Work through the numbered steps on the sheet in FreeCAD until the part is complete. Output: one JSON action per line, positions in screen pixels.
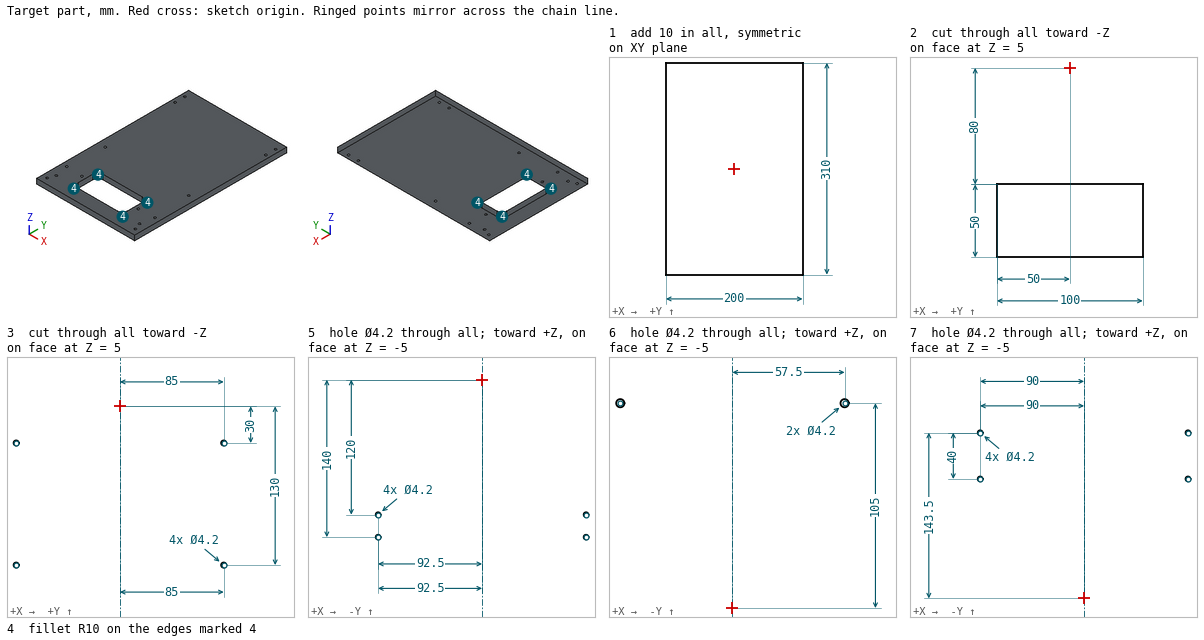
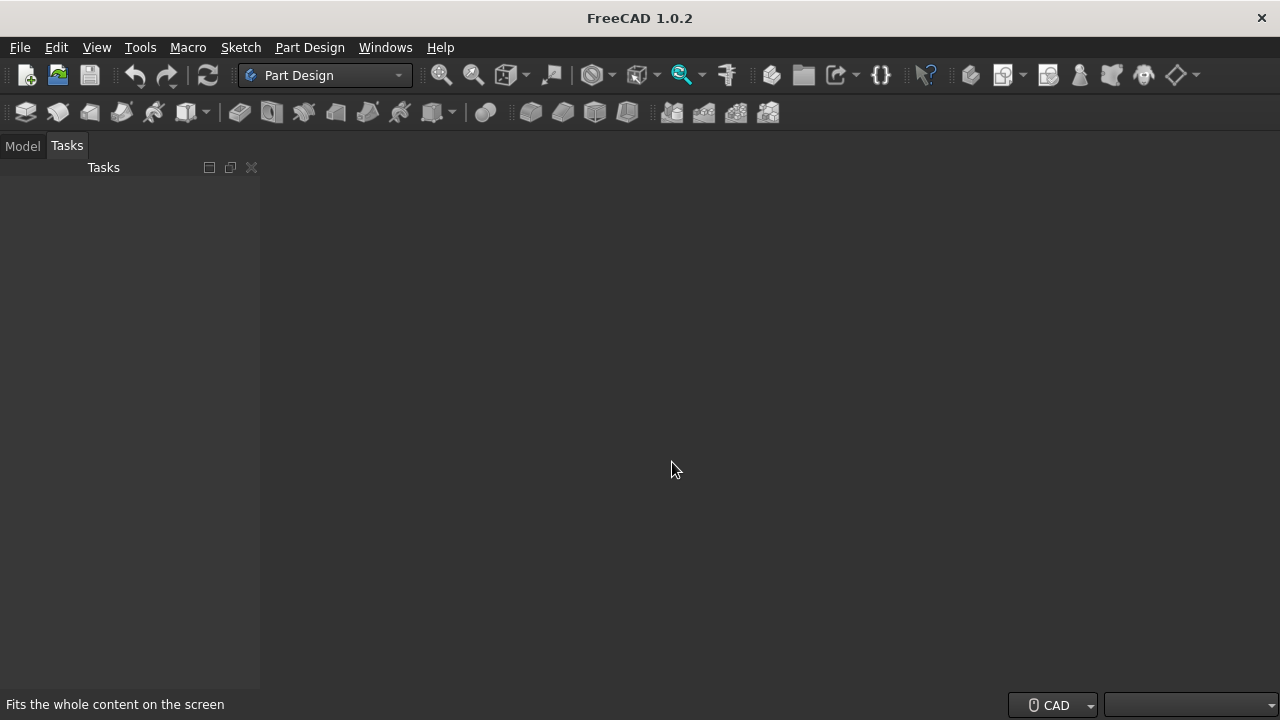
{"action": "left_click", "coordinate": [26, 76]}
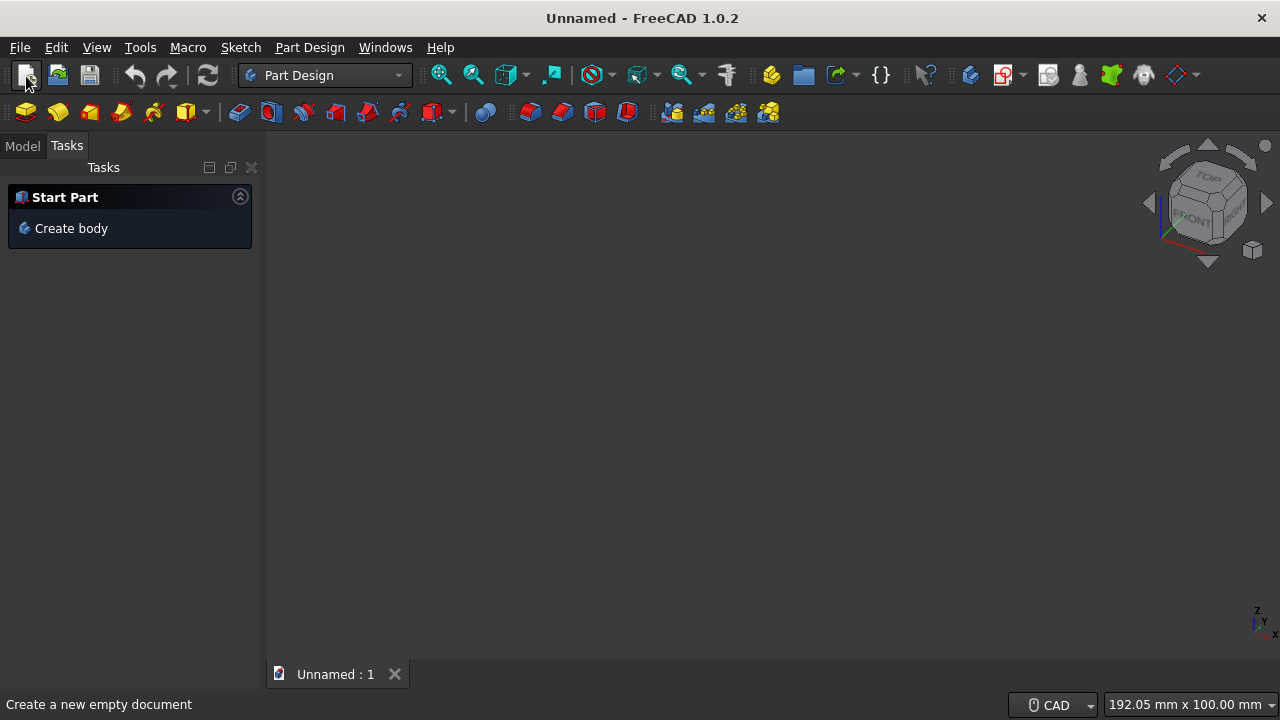
{"action": "left_click", "coordinate": [1004, 76]}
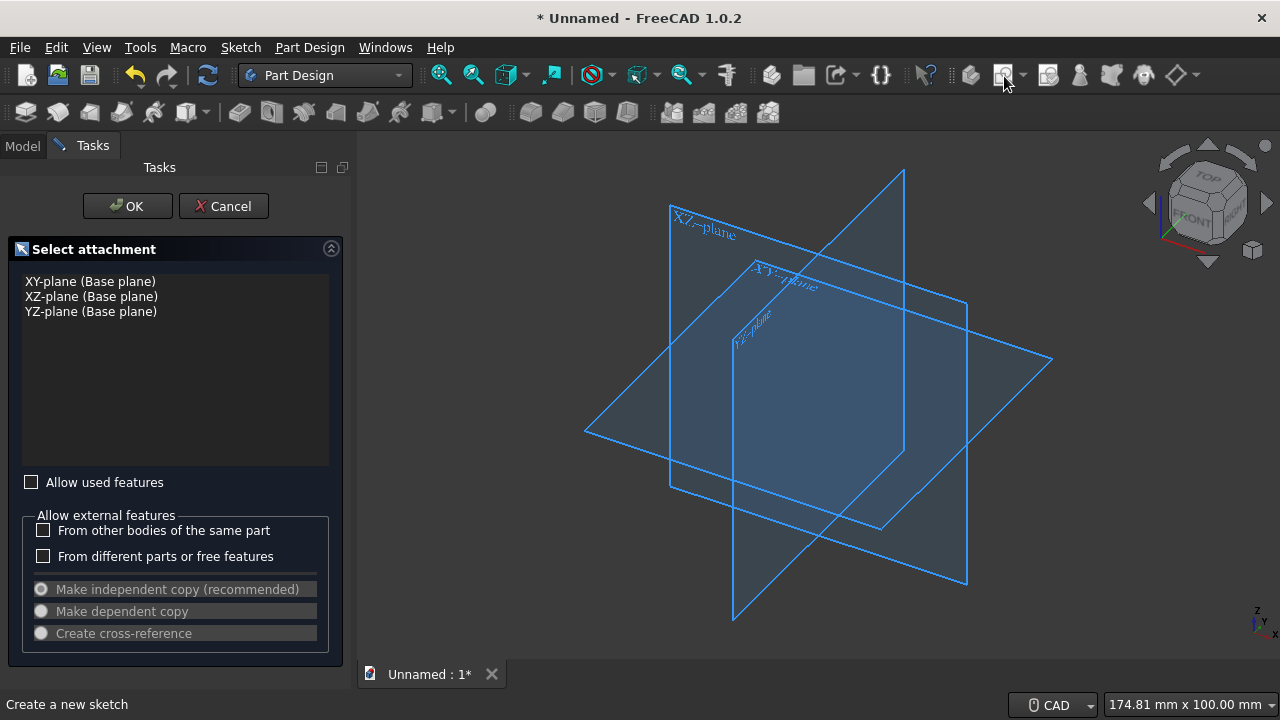
{"action": "left_click", "coordinate": [82, 282]}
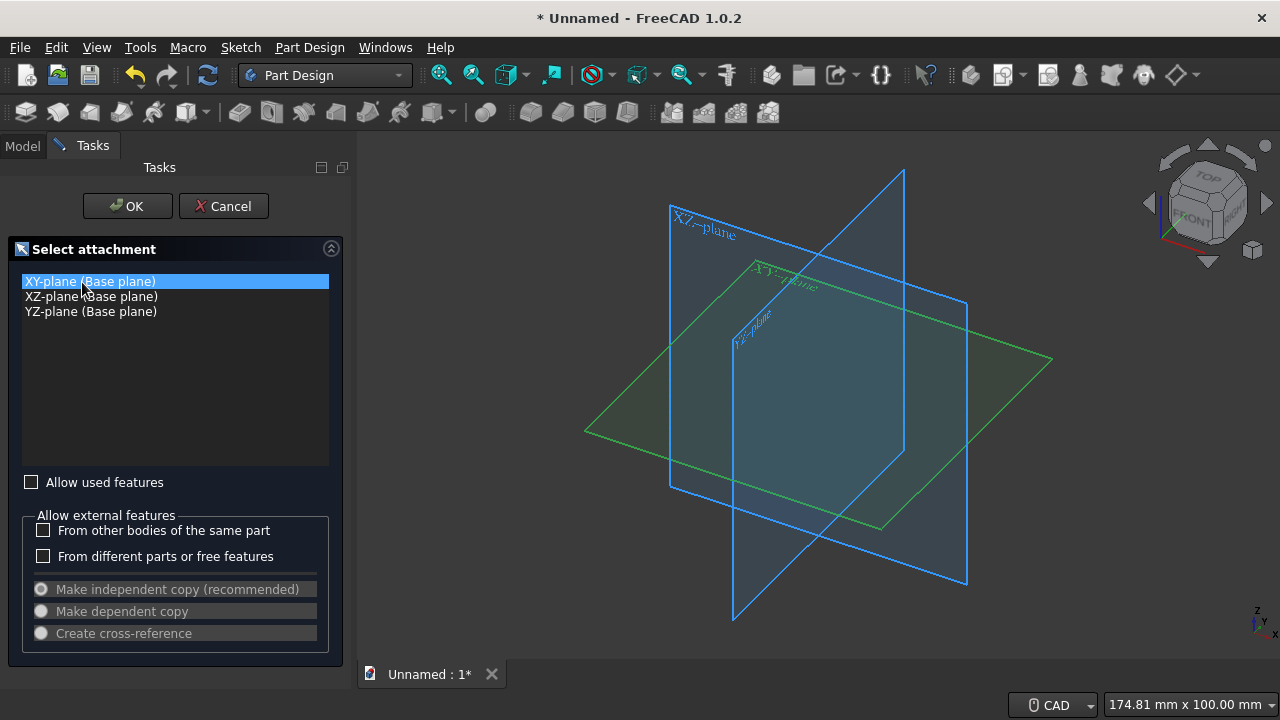
{"action": "left_click", "coordinate": [128, 206]}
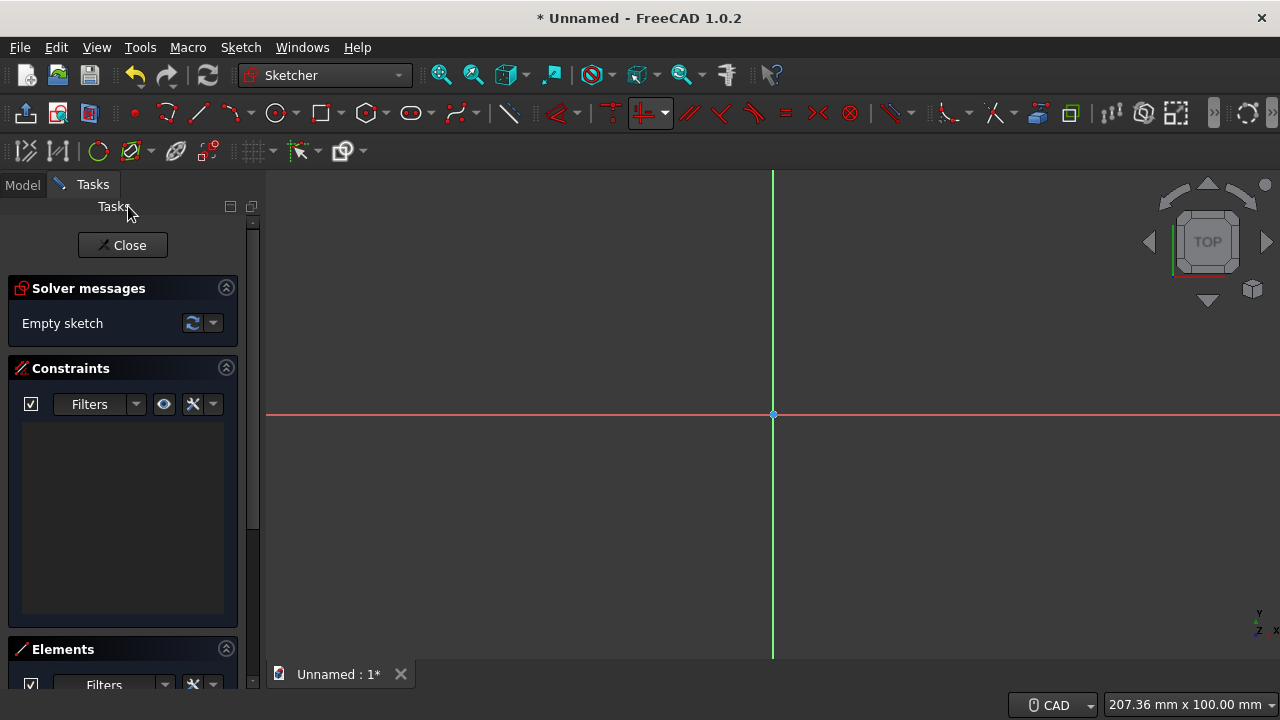
{"action": "scroll", "coordinate": [687, 414], "scroll_direction": "down", "scroll_amount": 8}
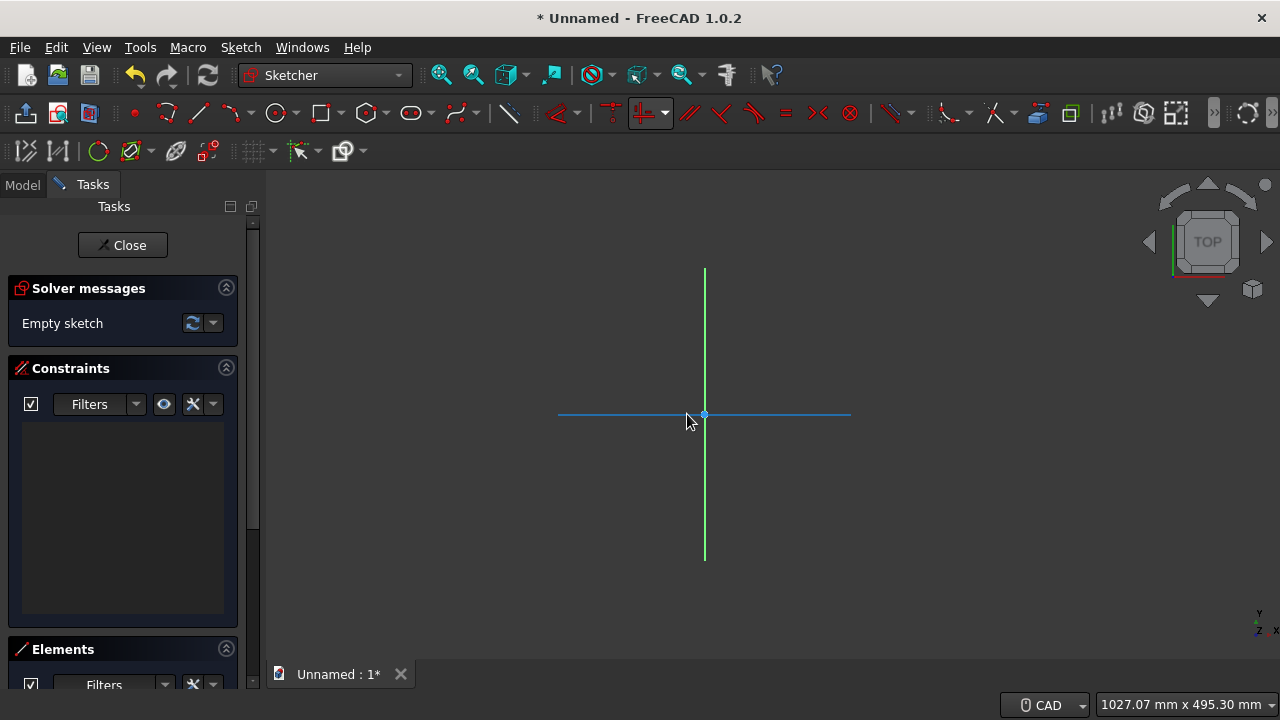
{"action": "key", "text": "g v"}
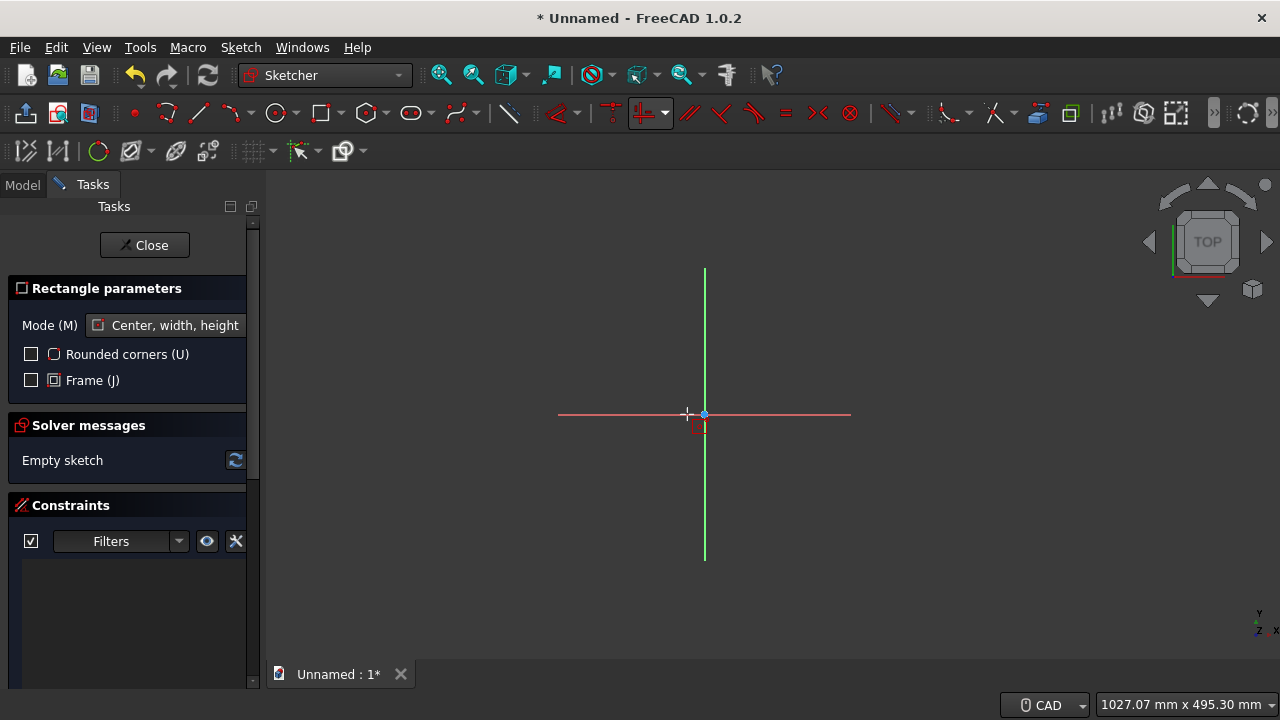
{"action": "left_click", "coordinate": [705, 414]}
{"action": "left_click", "coordinate": [803, 261]}
{"action": "key", "text": "Escape"}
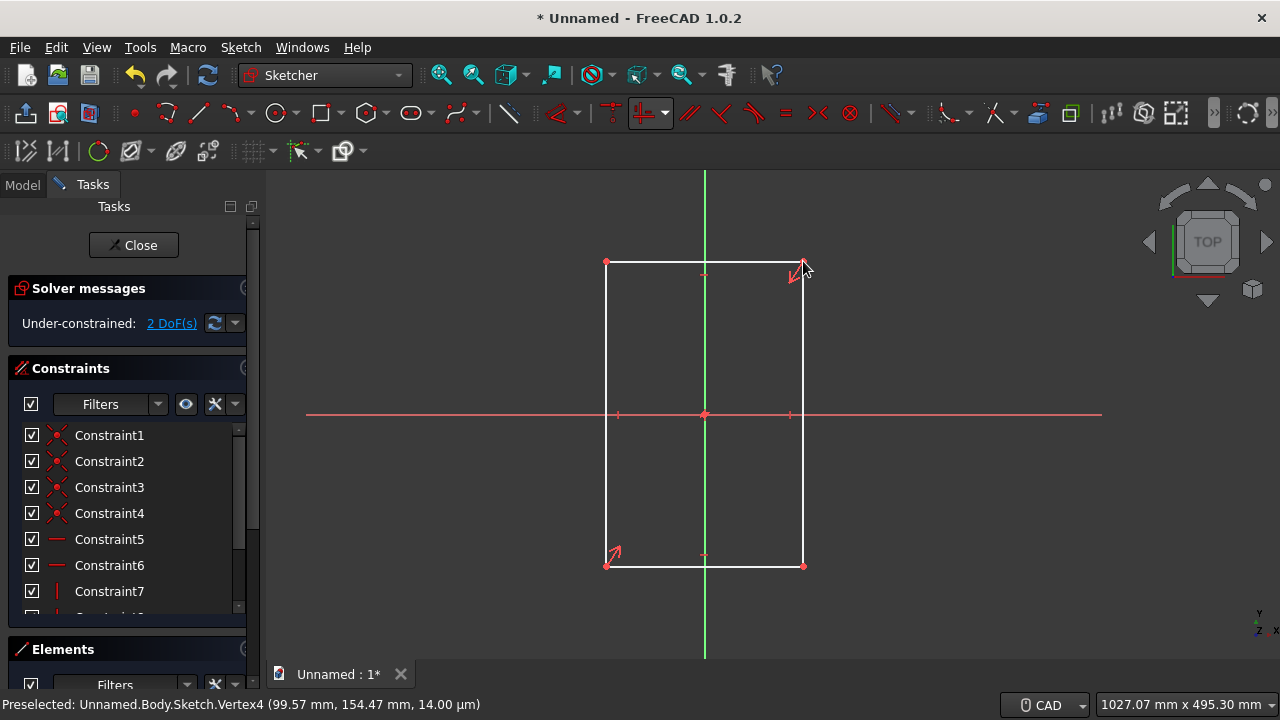
{"action": "left_click", "coordinate": [556, 114]}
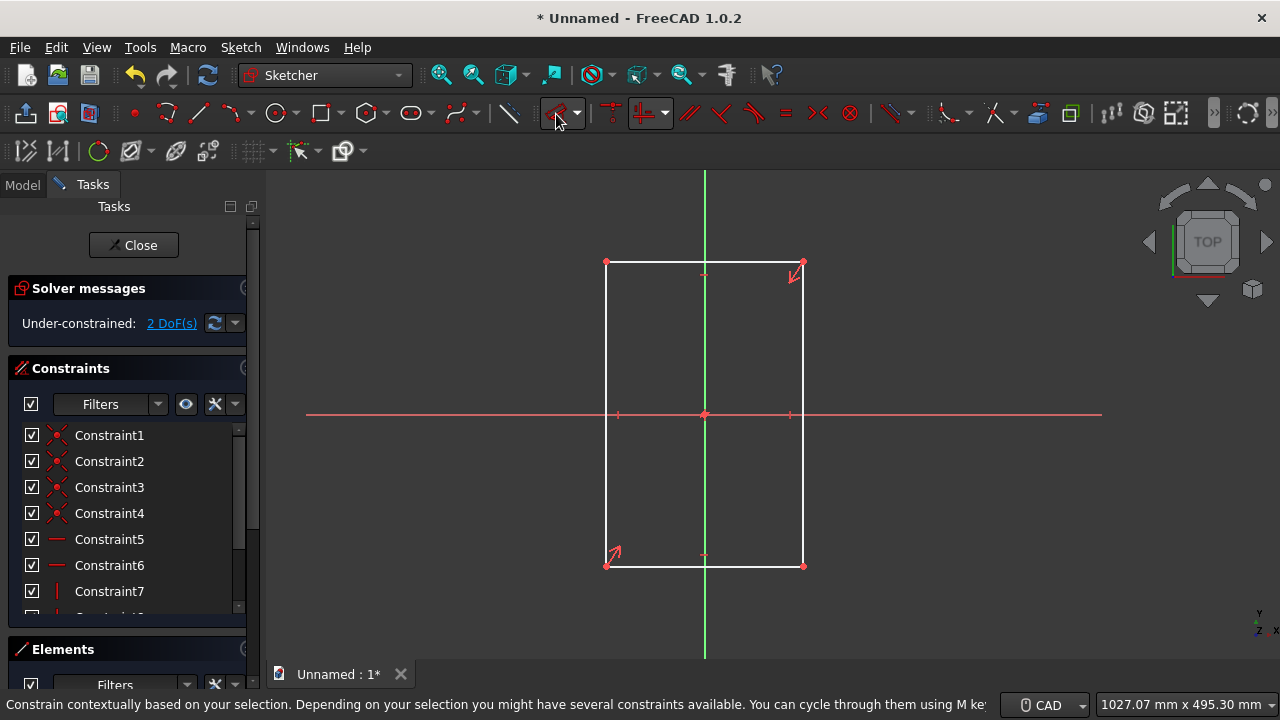
{"action": "left_click", "coordinate": [665, 567]}
{"action": "left_click", "coordinate": [659, 601]}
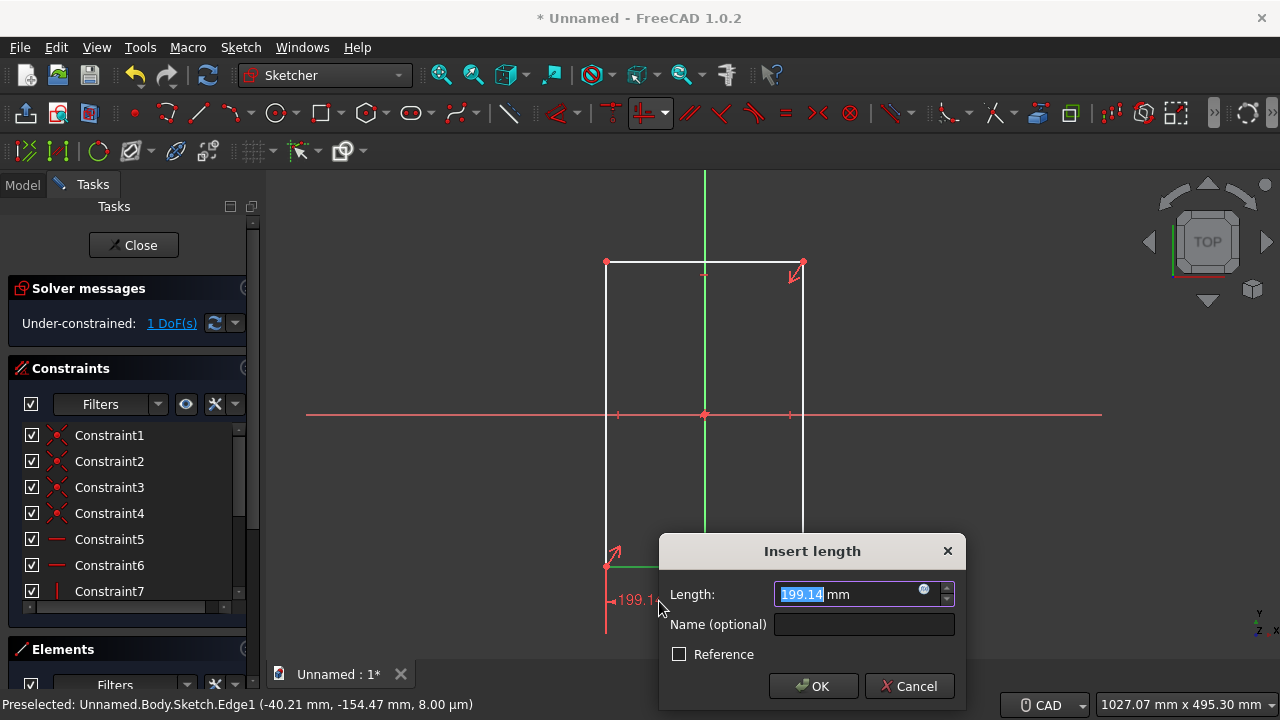
{"action": "type", "text": "200"}
{"action": "key", "text": "Return"}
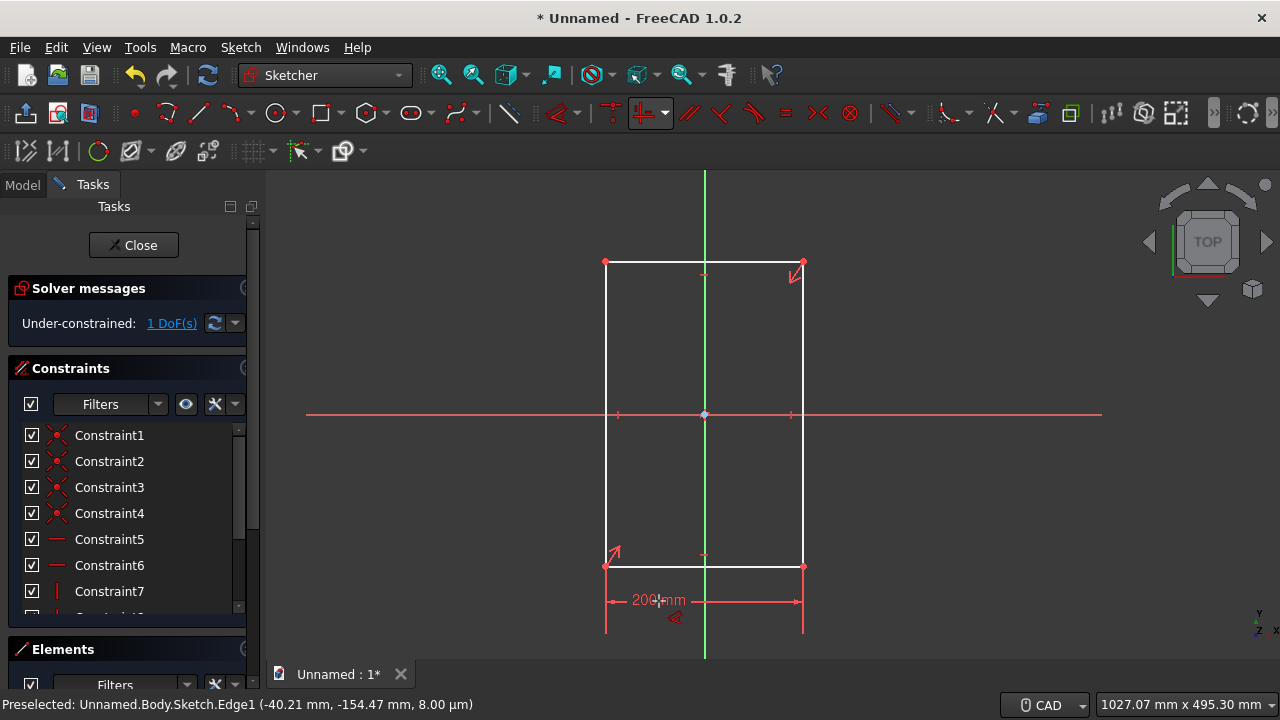
{"action": "left_click", "coordinate": [803, 475]}
{"action": "left_click", "coordinate": [837, 344]}